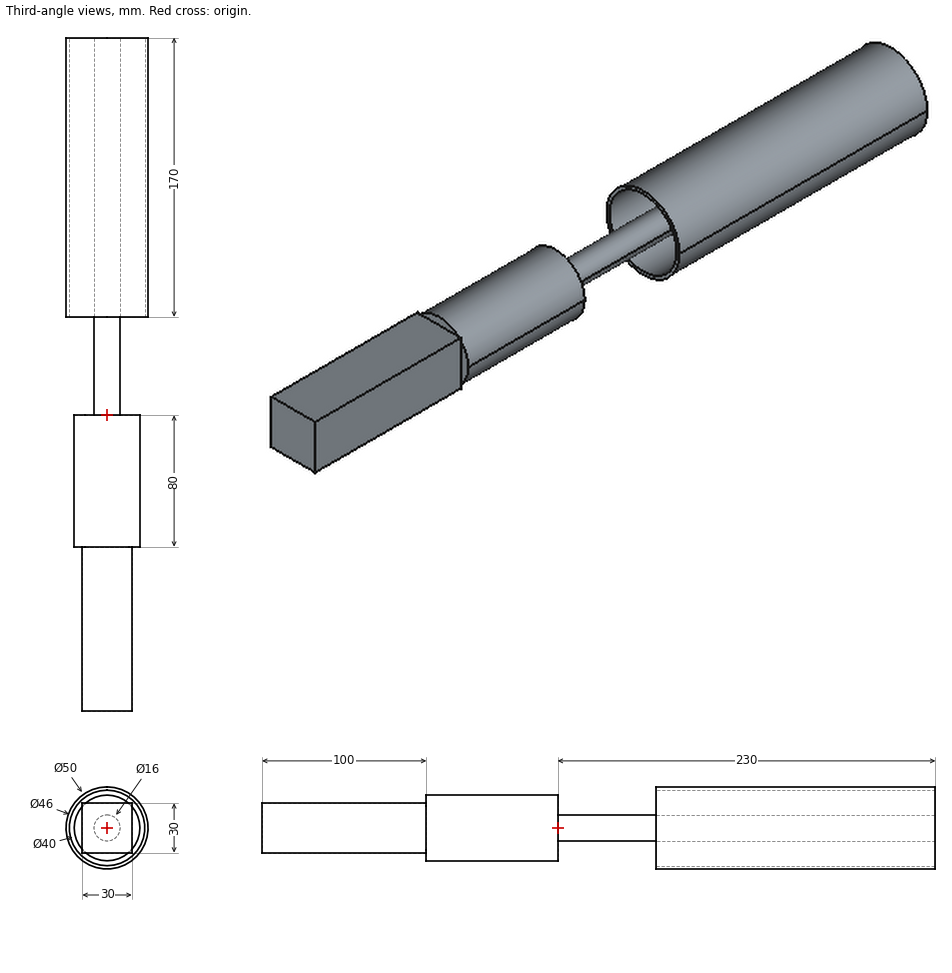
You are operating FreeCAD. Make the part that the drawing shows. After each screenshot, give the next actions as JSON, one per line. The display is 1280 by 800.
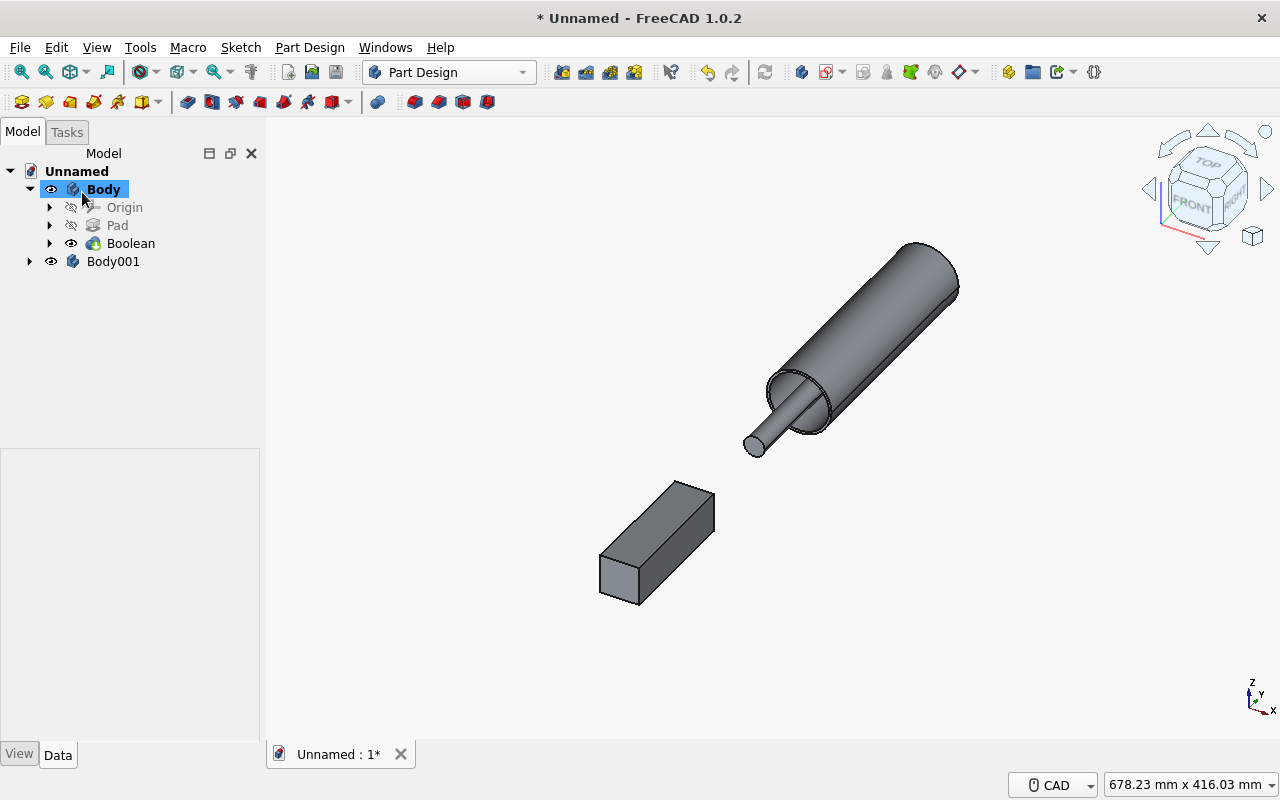
{"action": "left_click", "coordinate": [826, 72]}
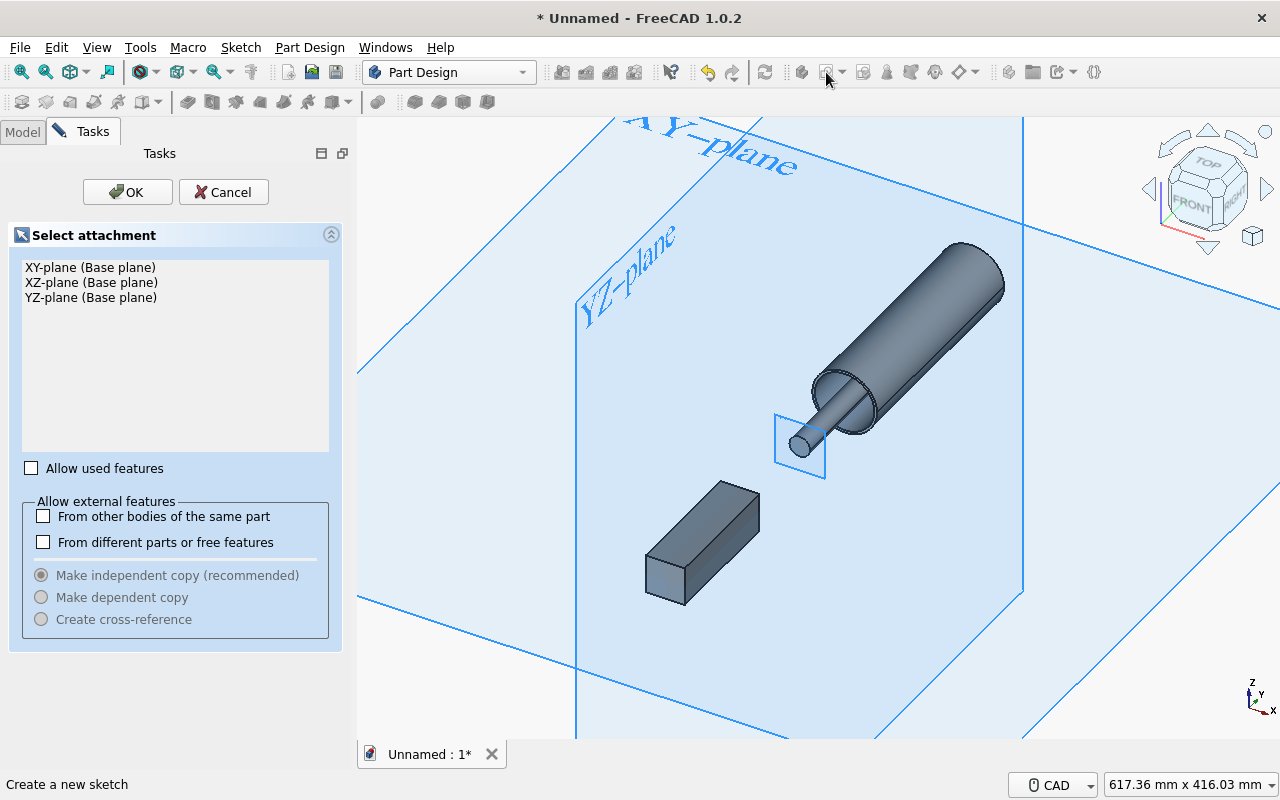
{"action": "left_click", "coordinate": [82, 282]}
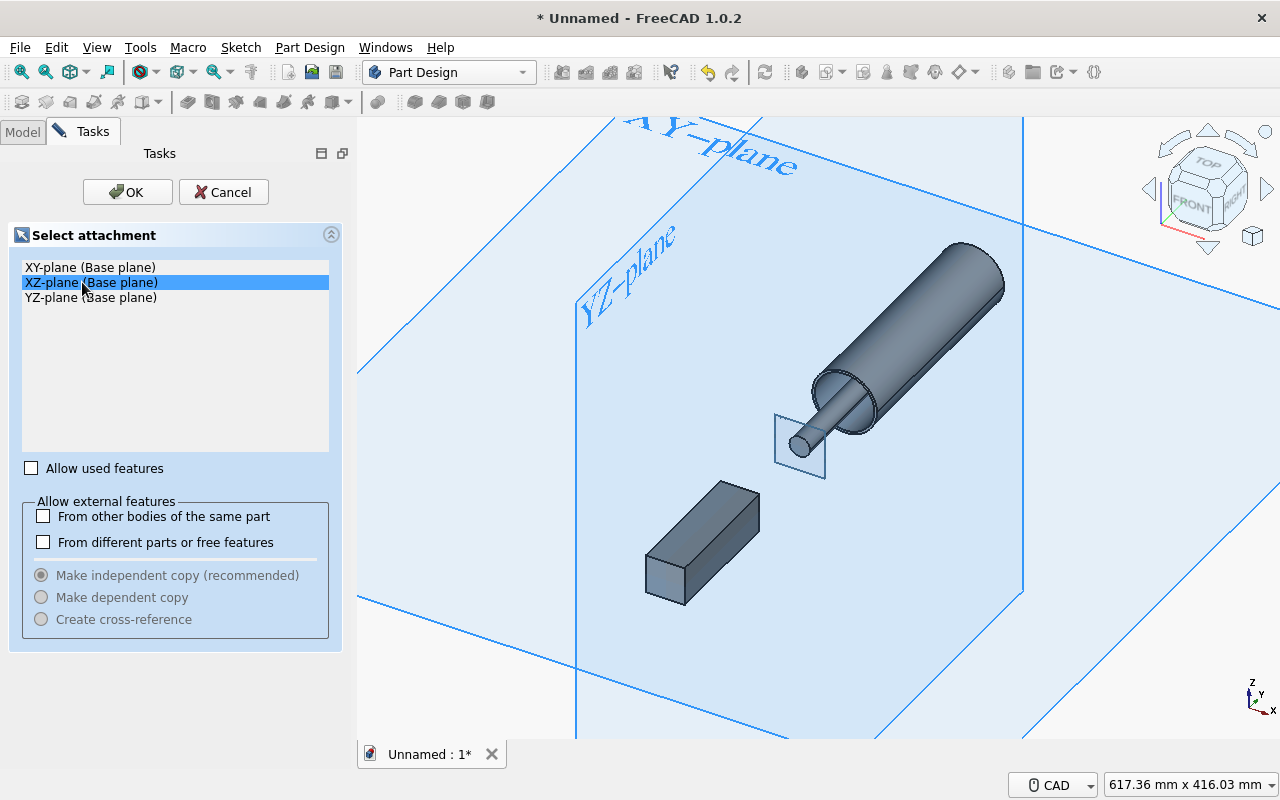
{"action": "left_click", "coordinate": [128, 192]}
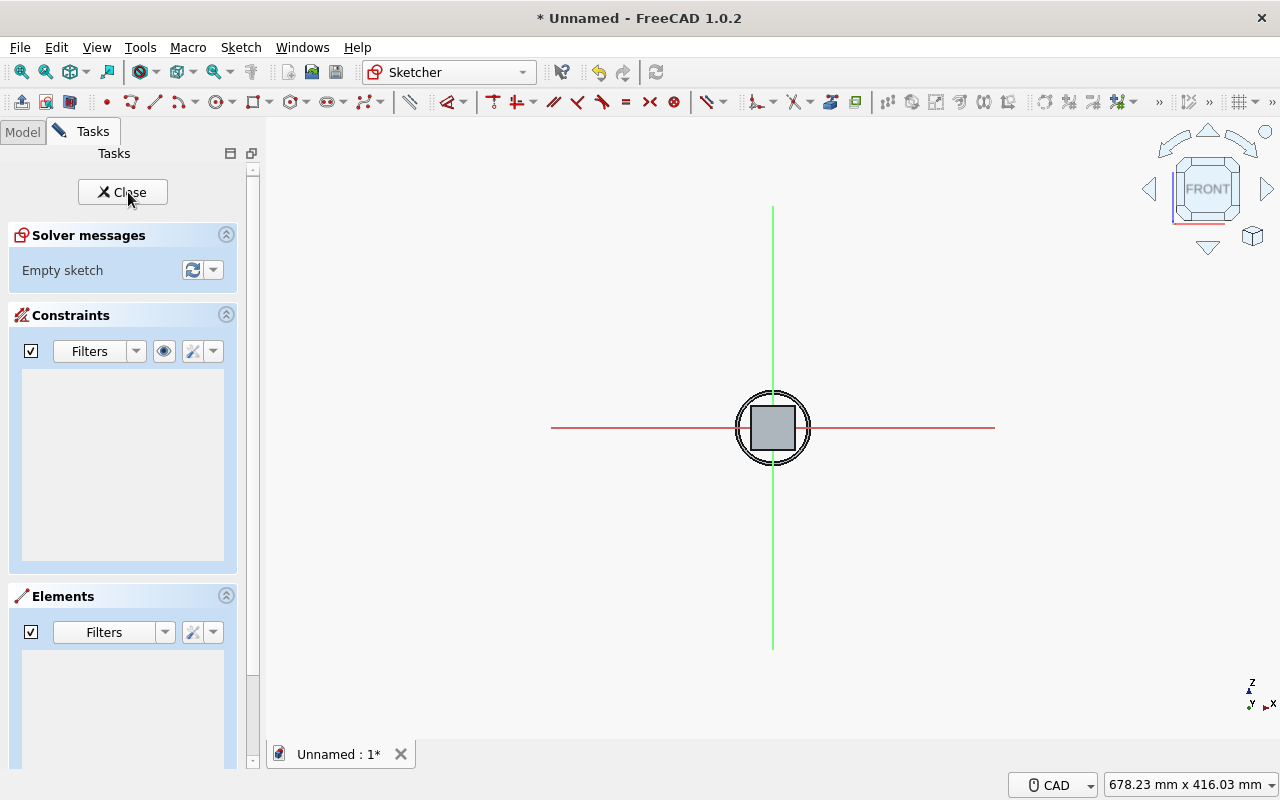
{"action": "left_click", "coordinate": [70, 102]}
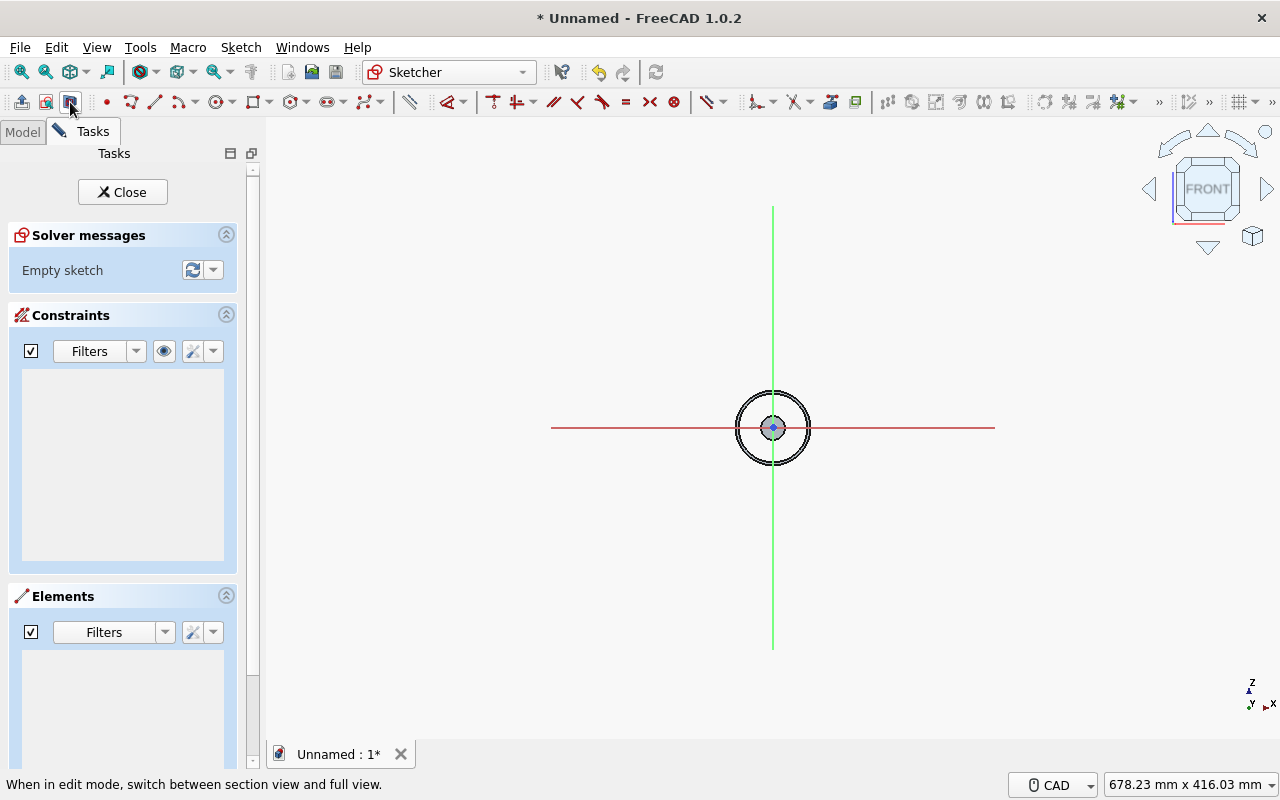
{"action": "scroll", "coordinate": [787, 428], "scroll_direction": "up", "scroll_amount": 9}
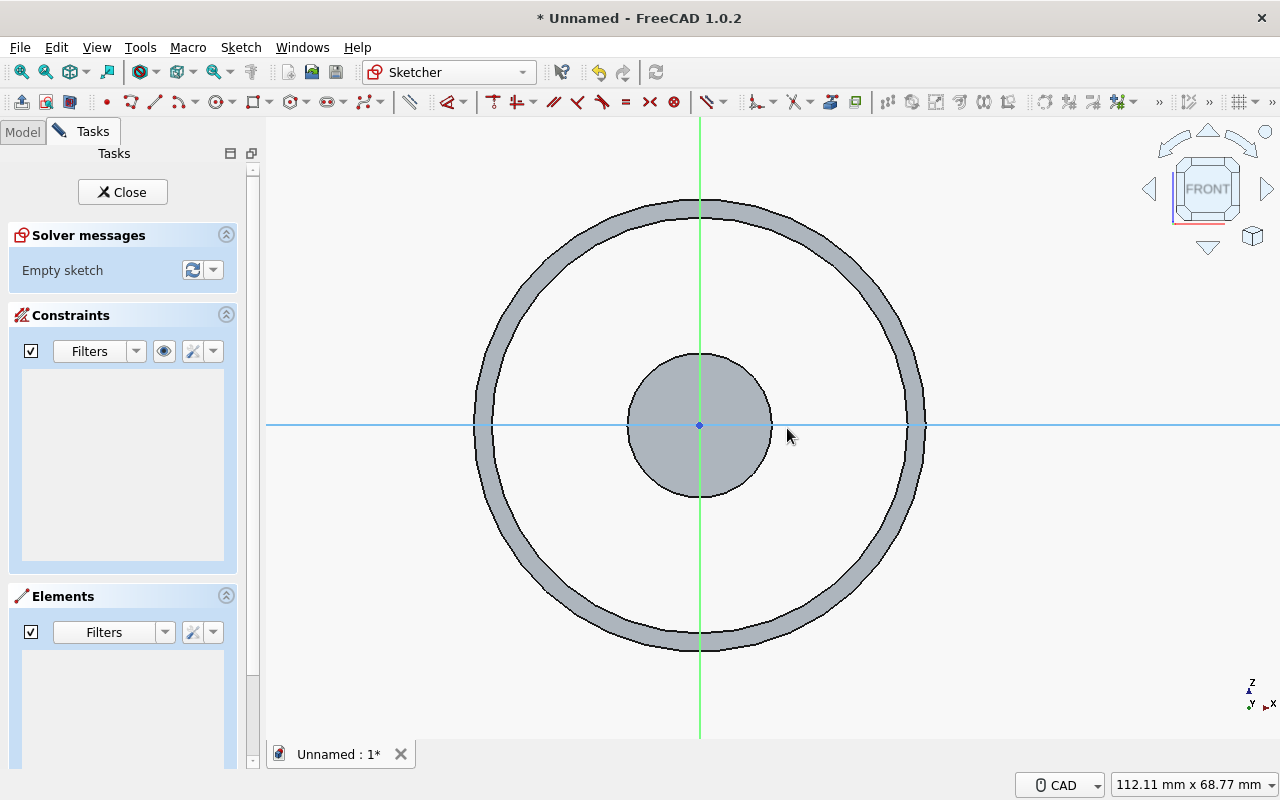
{"action": "left_click", "coordinate": [216, 102]}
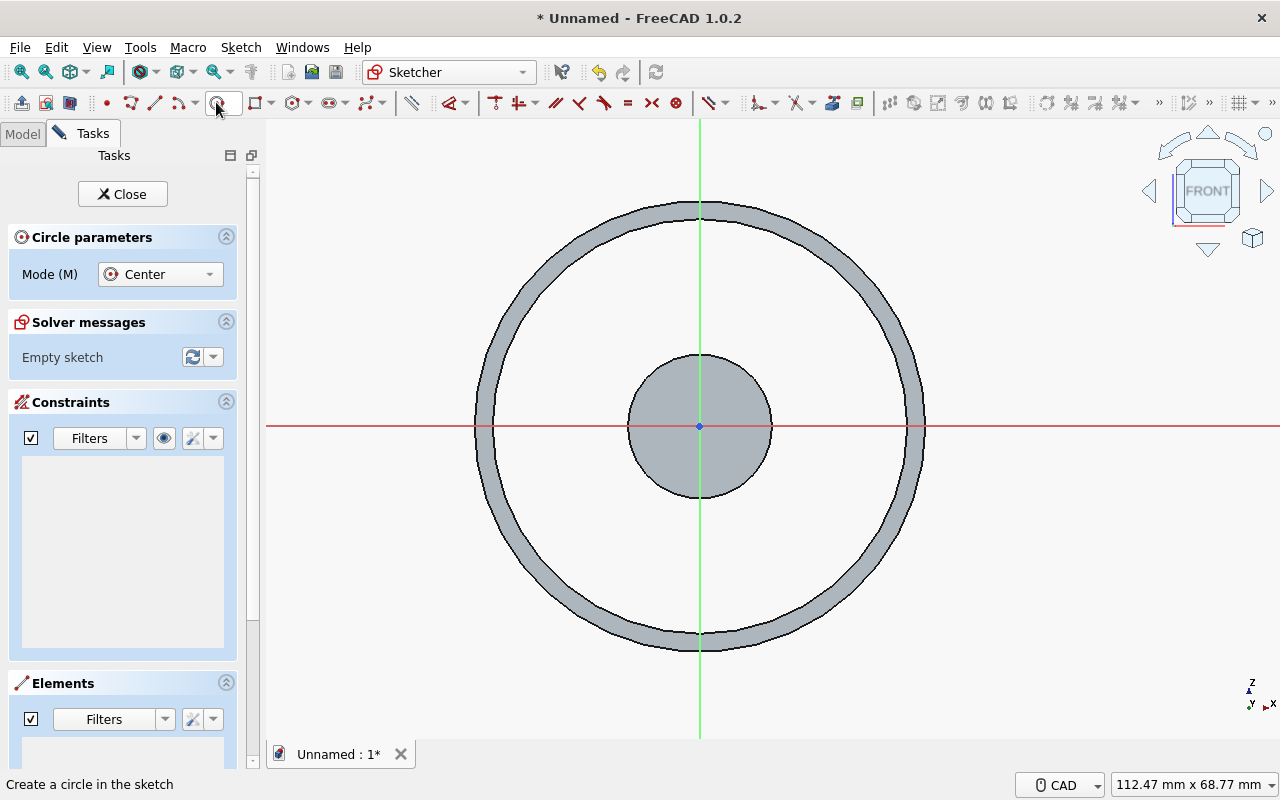
{"action": "left_click", "coordinate": [700, 426]}
{"action": "mouse_move", "coordinate": [827, 299]}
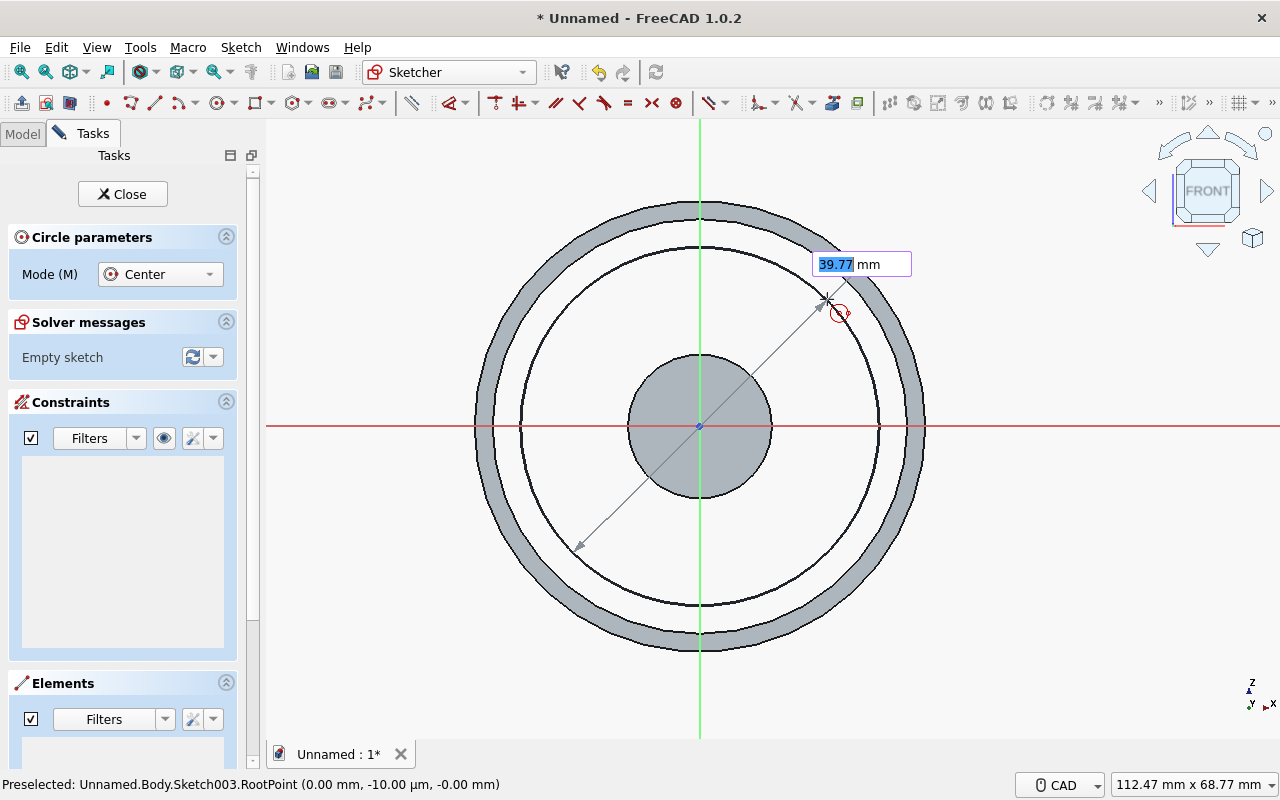
{"action": "type", "text": "40"}
{"action": "key", "text": "Return"}
{"action": "key", "text": "Escape"}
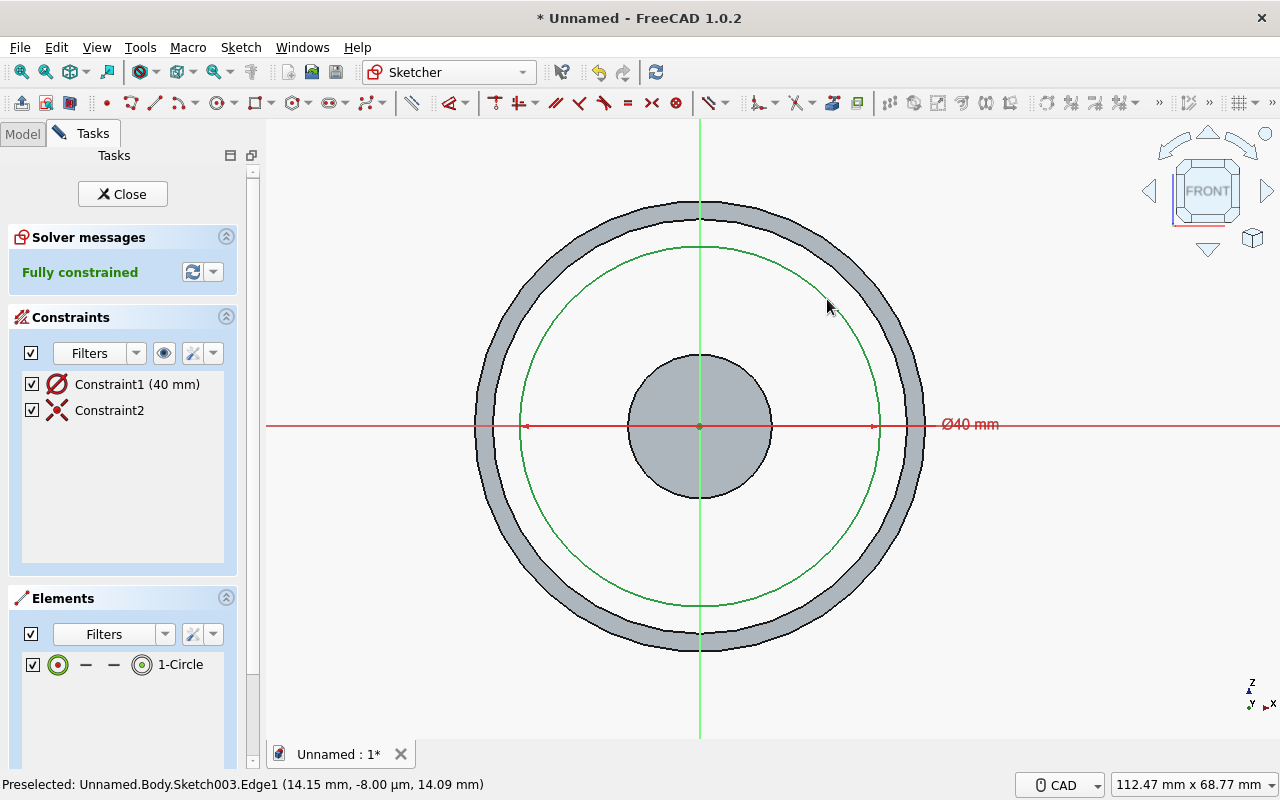
{"action": "left_click", "coordinate": [123, 194]}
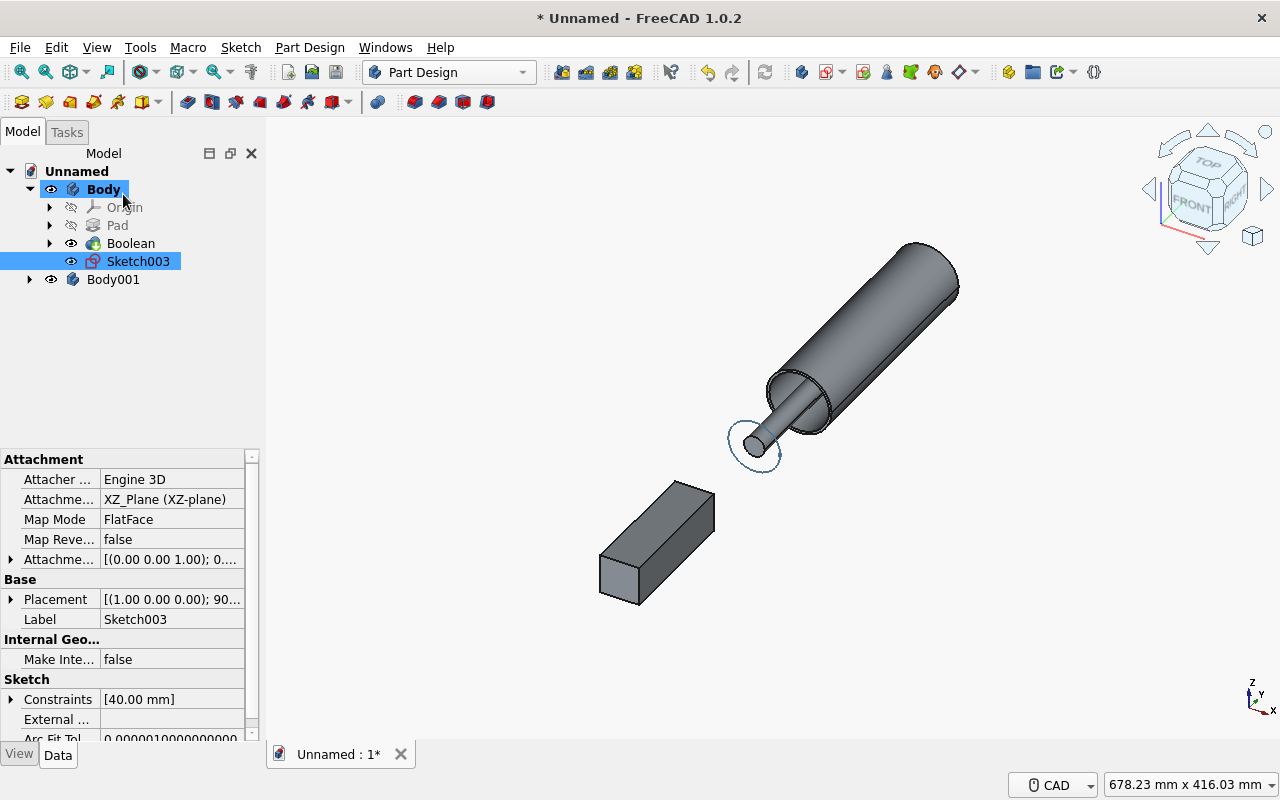
{"action": "left_click", "coordinate": [22, 102]}